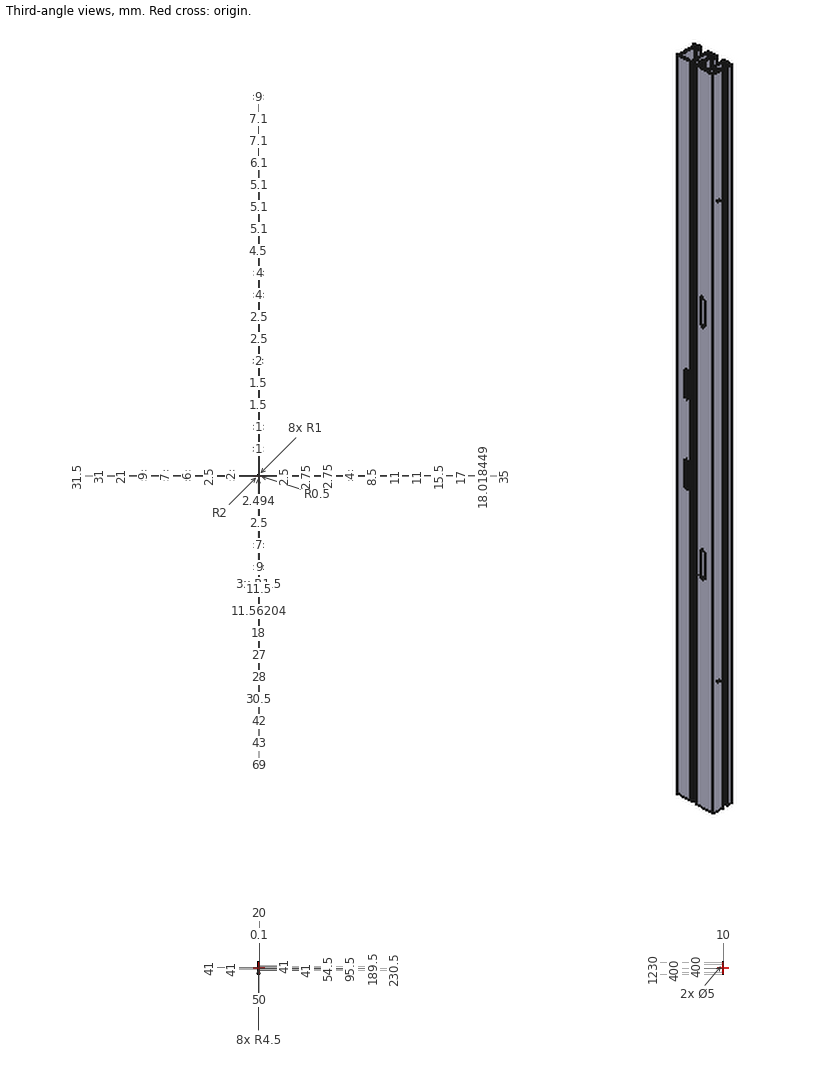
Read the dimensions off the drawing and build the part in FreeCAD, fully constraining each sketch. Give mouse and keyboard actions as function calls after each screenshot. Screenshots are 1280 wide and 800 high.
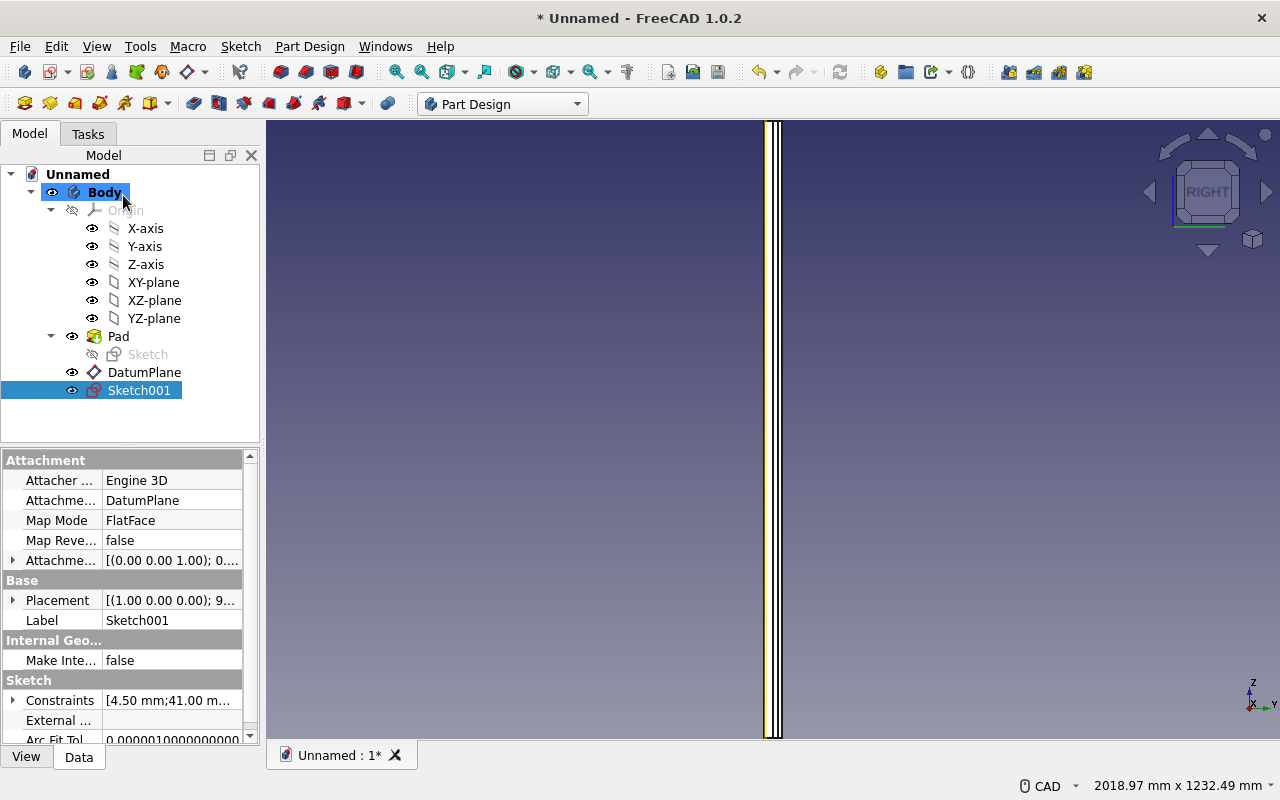
click(194, 104)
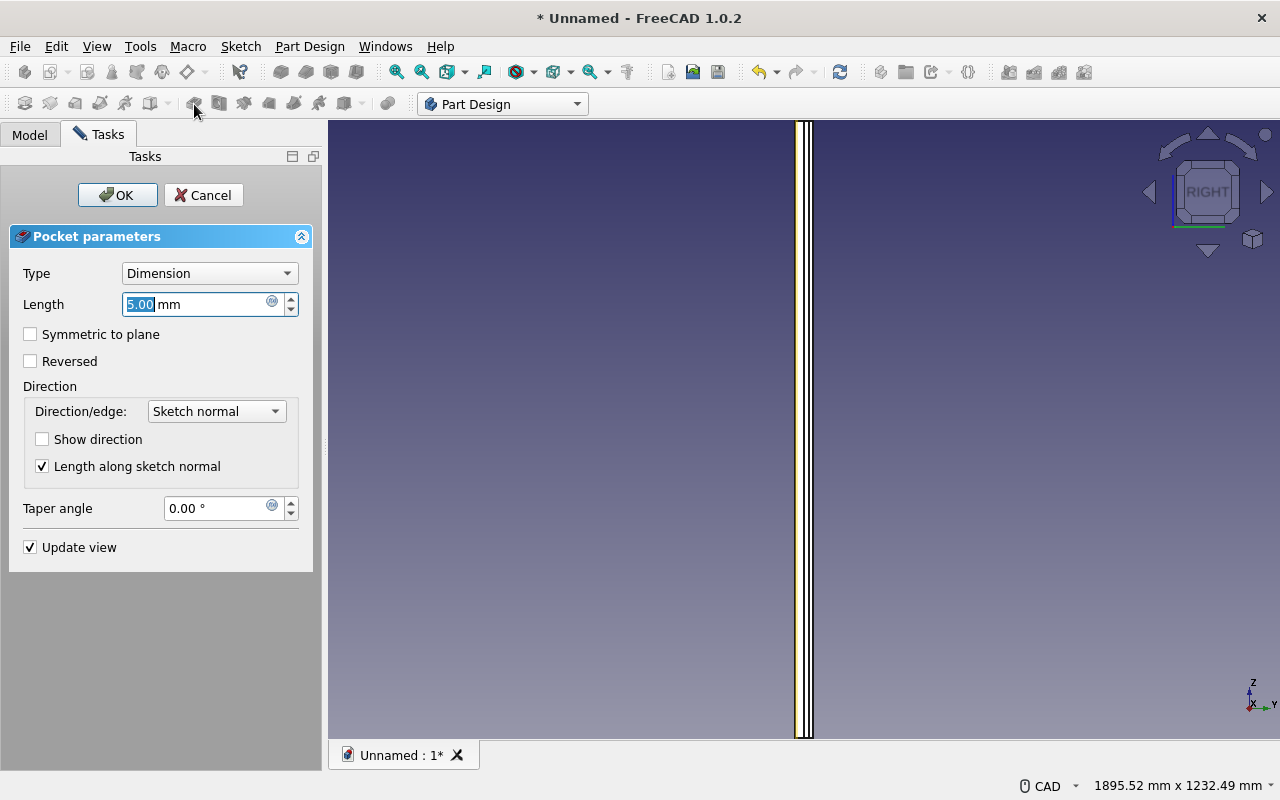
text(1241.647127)
key(Tab)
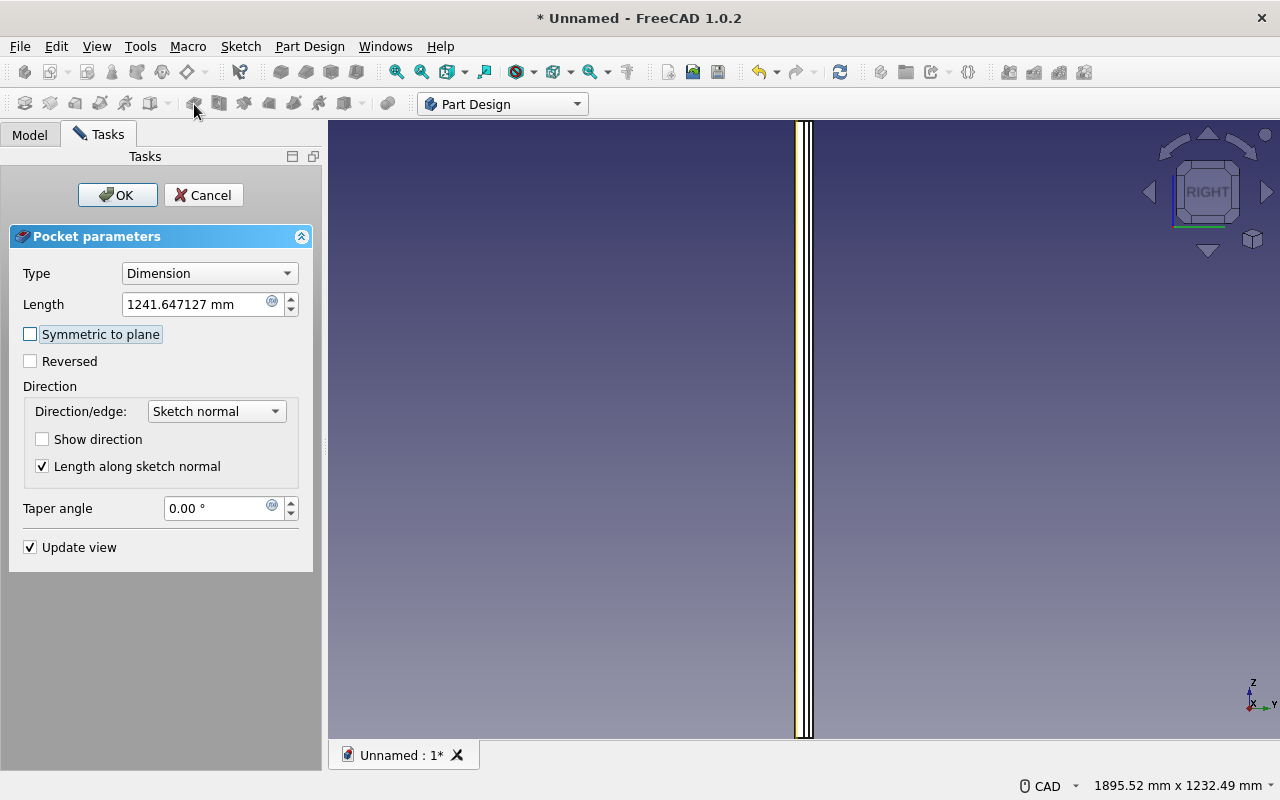
click(31, 334)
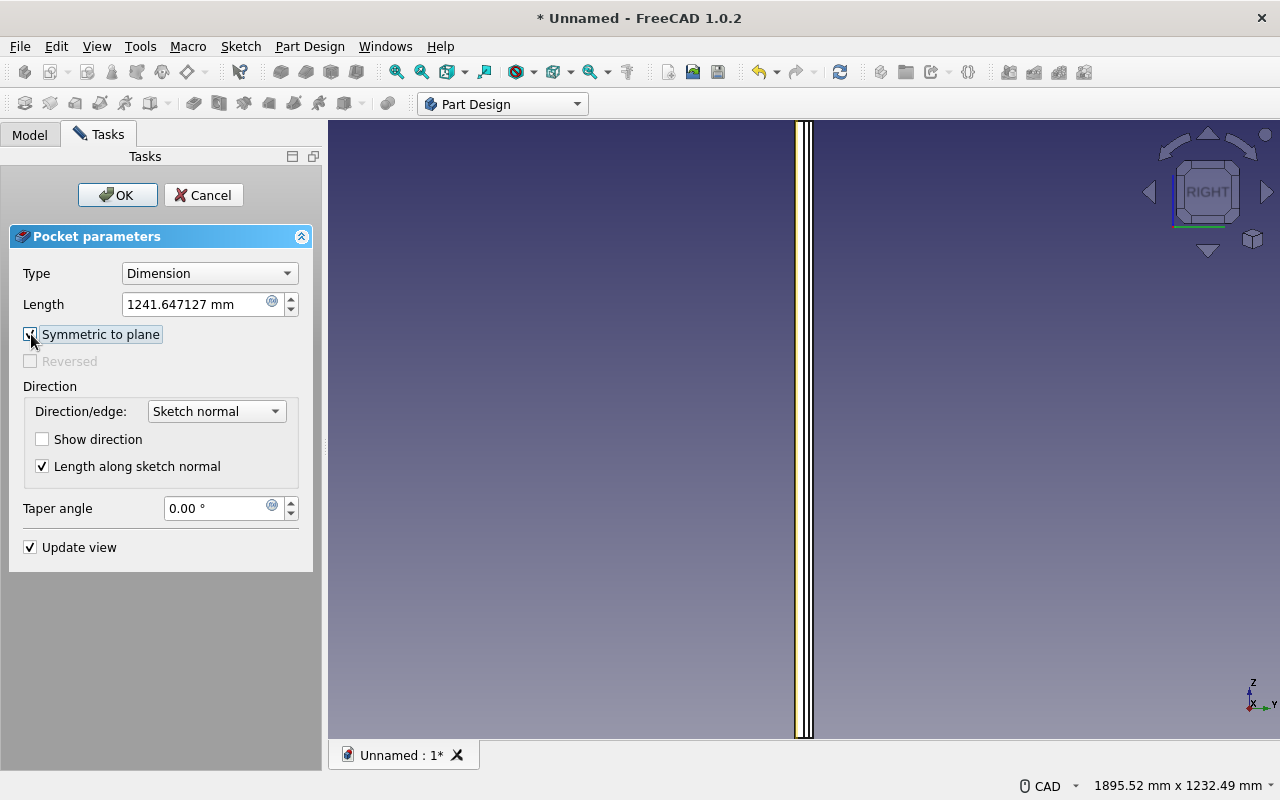
click(118, 195)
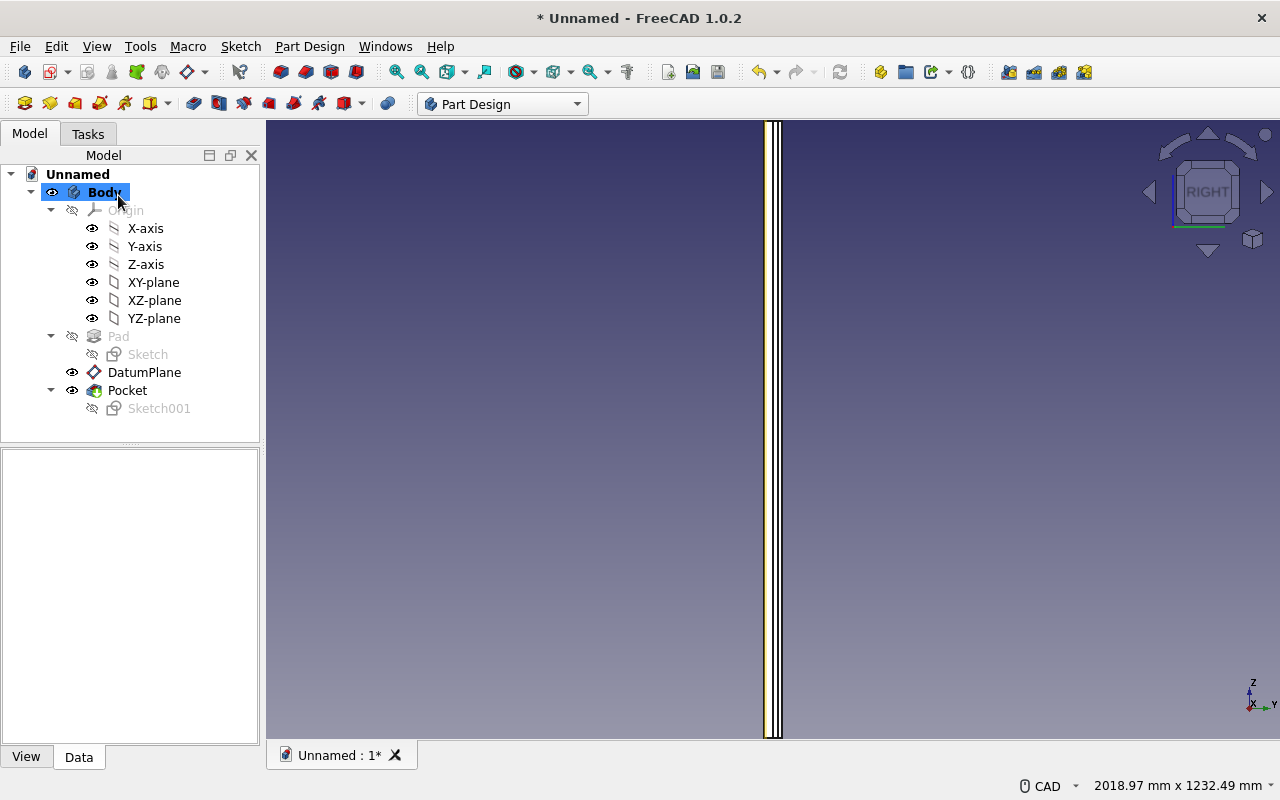
click(117, 372)
key(space)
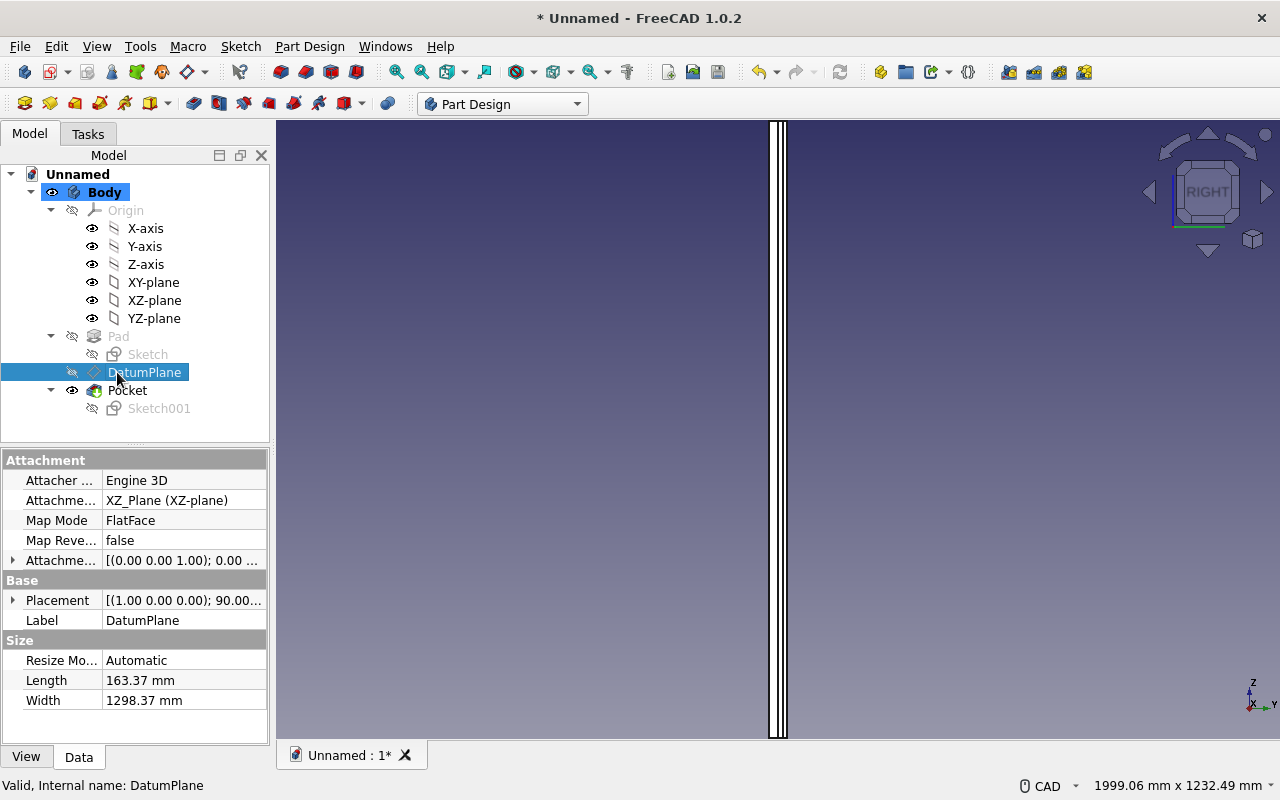
click(316, 699)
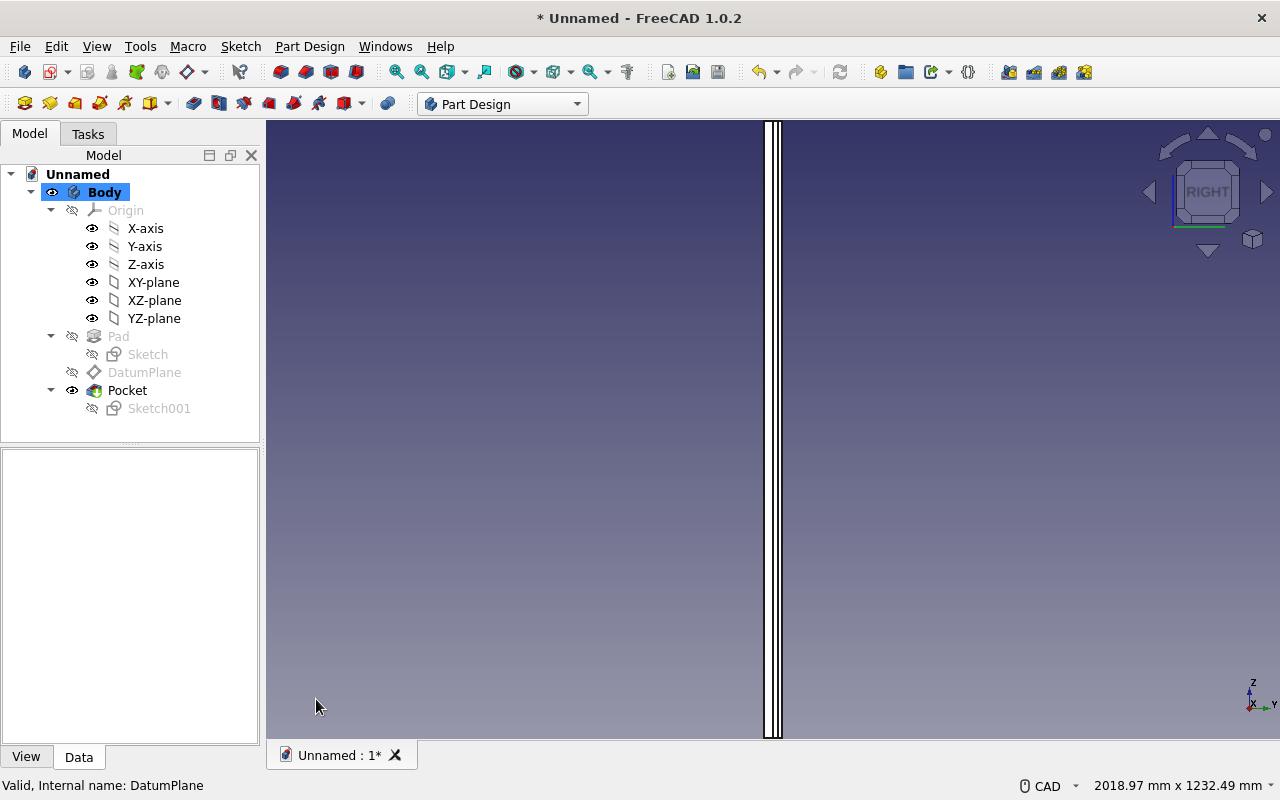
click(50, 72)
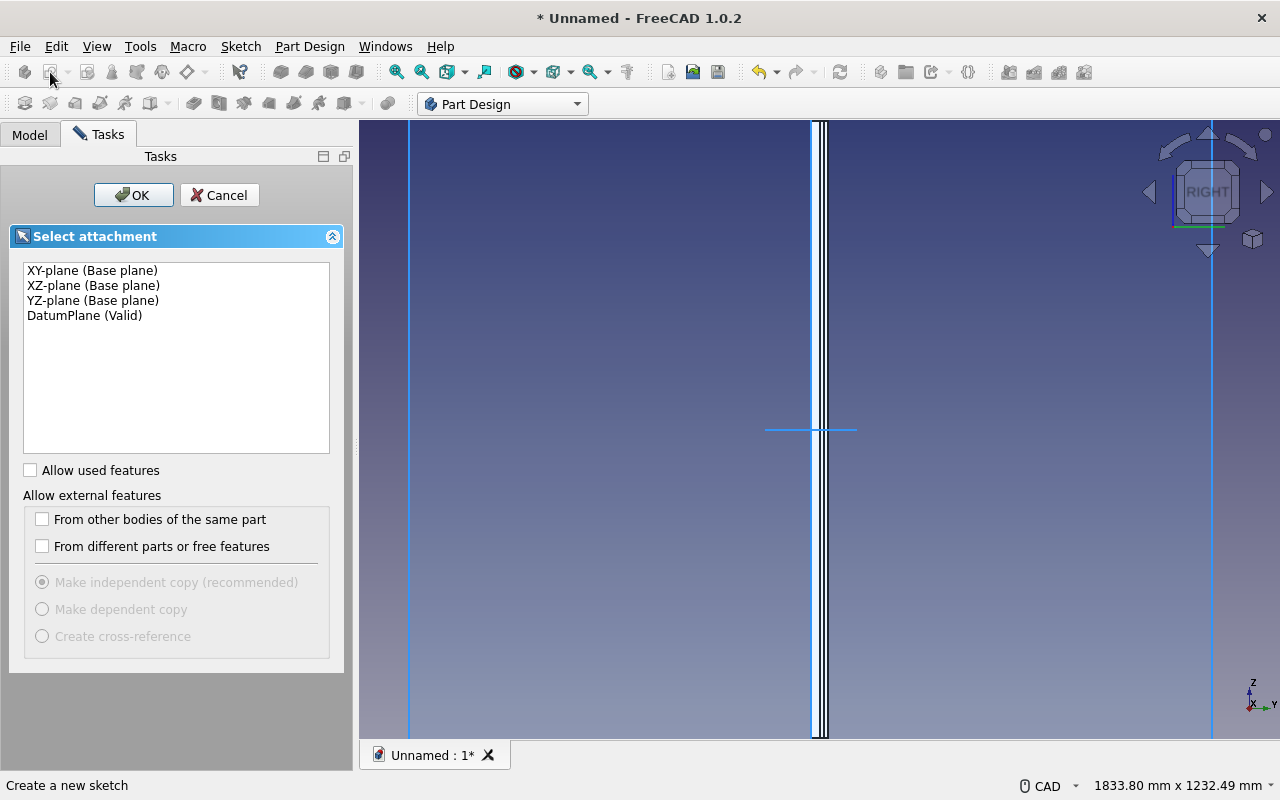
click(84, 300)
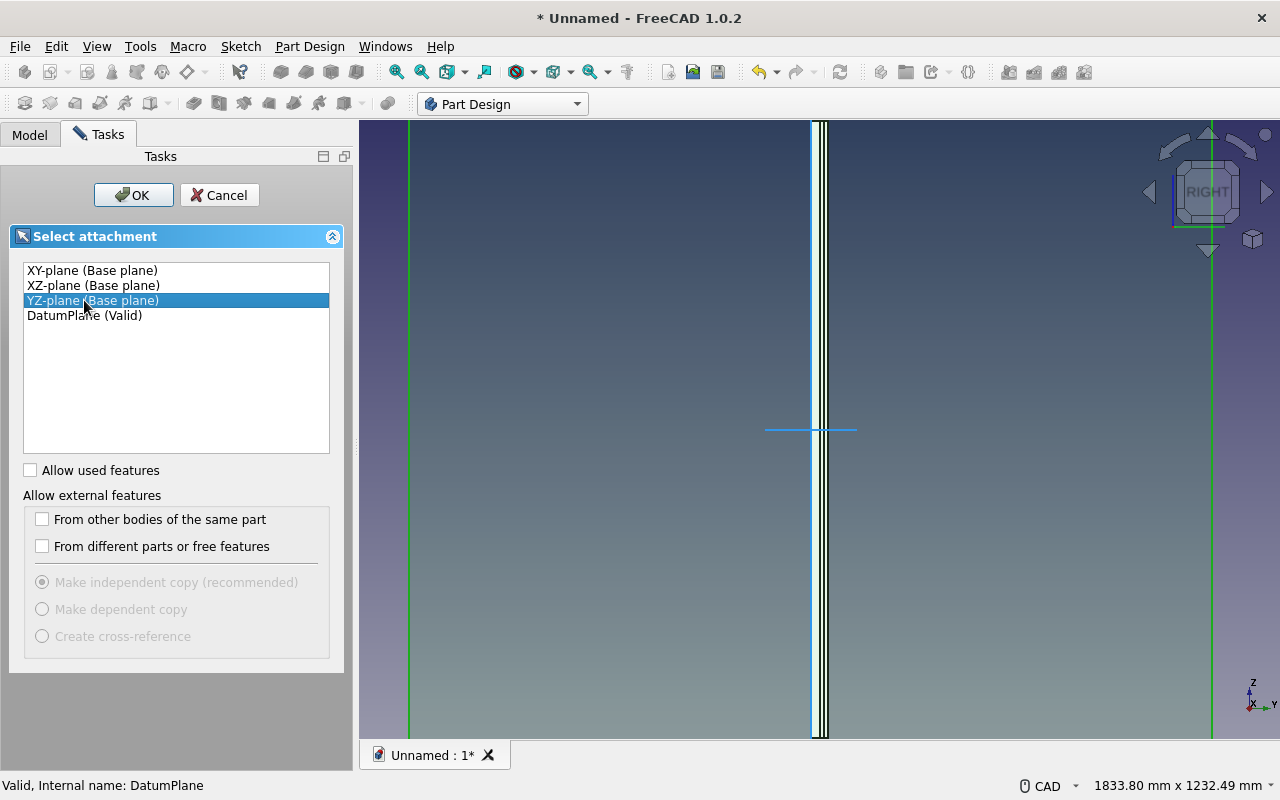
click(134, 195)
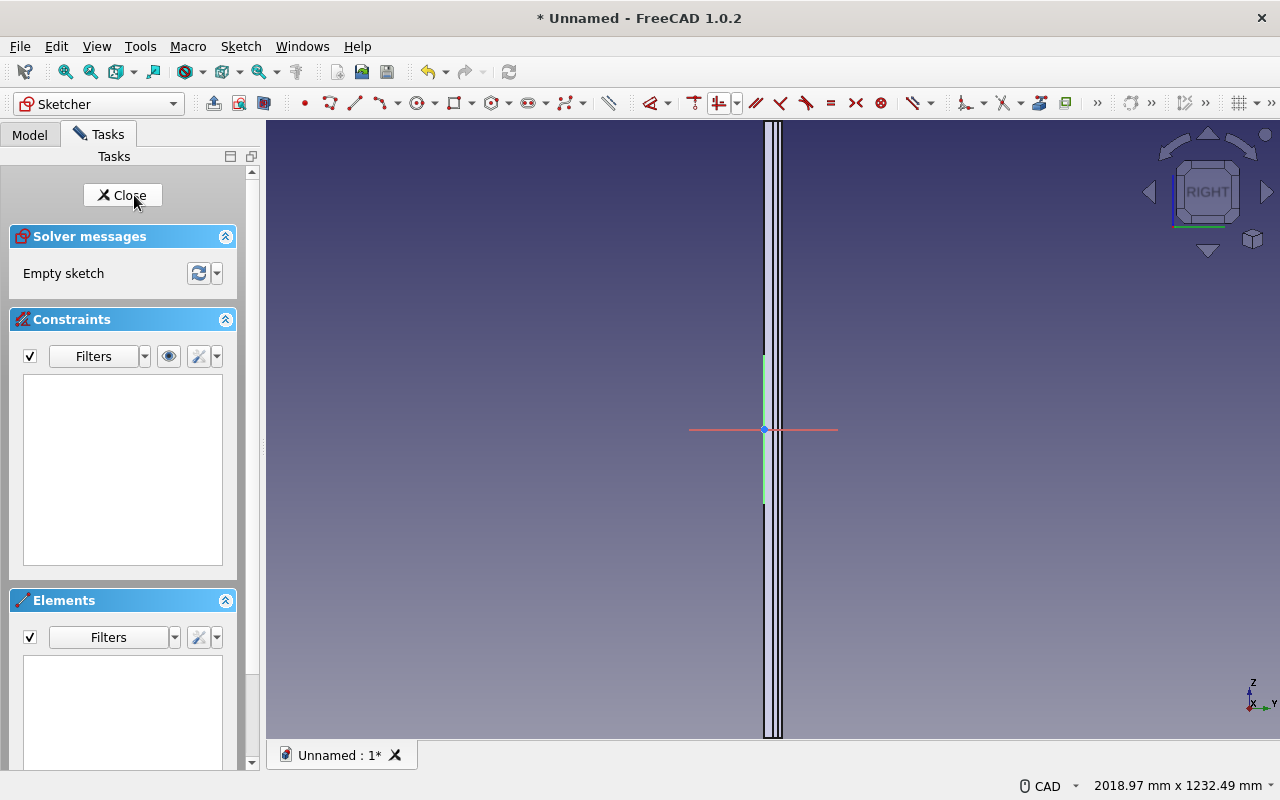
click(416, 104)